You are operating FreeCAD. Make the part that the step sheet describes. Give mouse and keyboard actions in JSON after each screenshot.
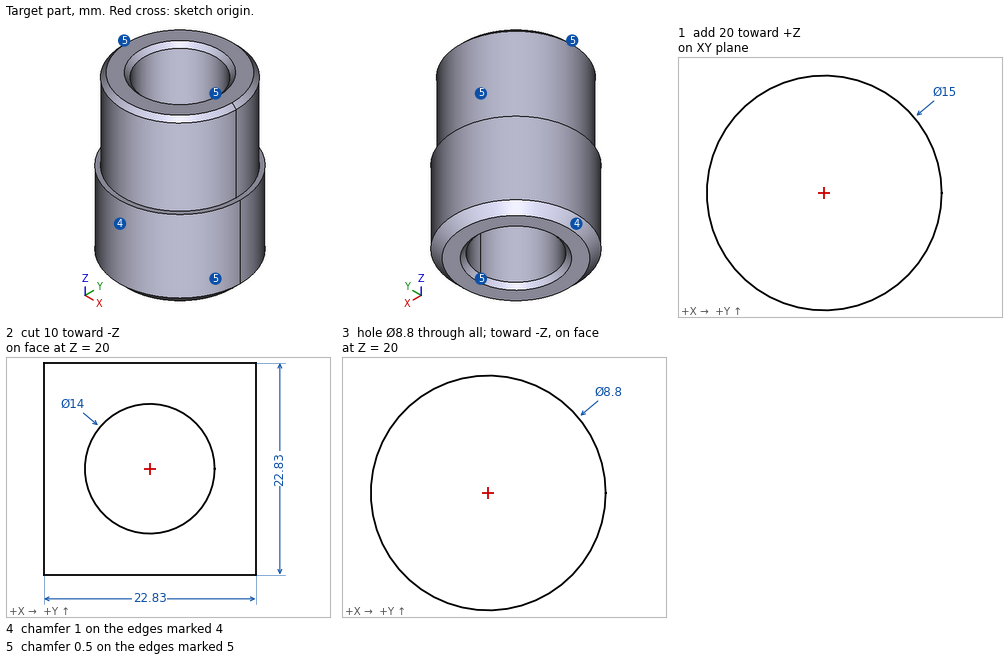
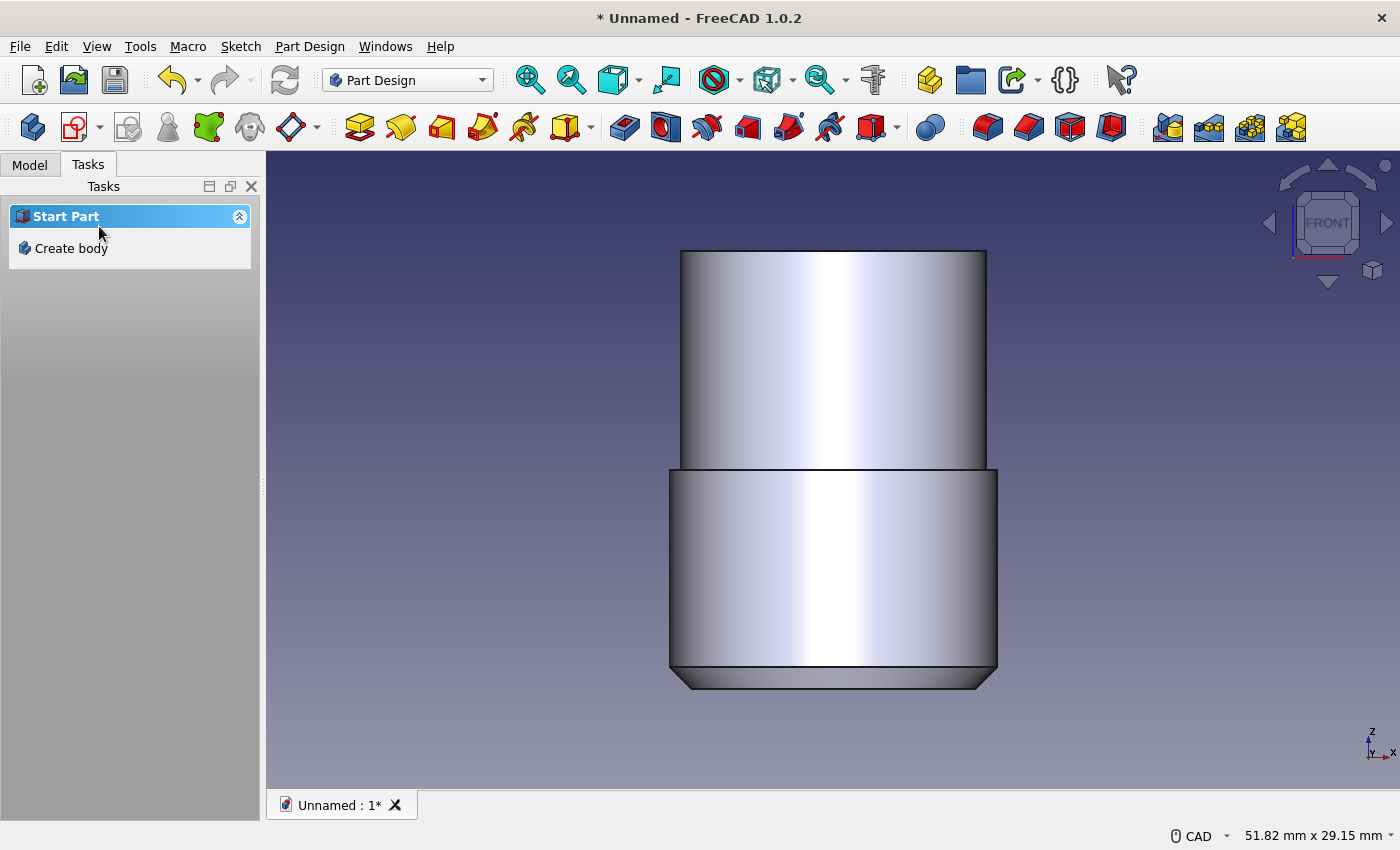
{"action": "left_click", "coordinate": [709, 250]}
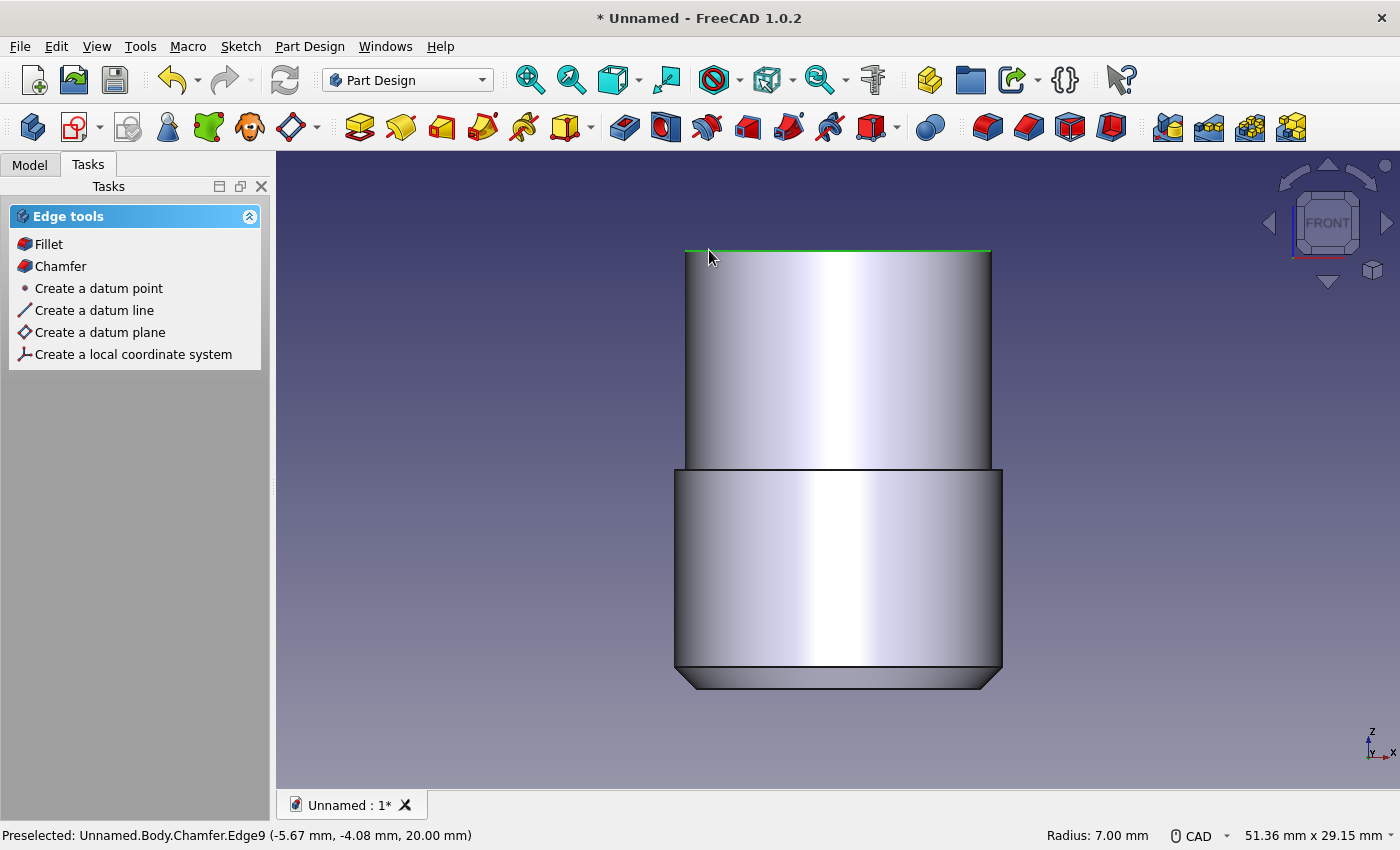
{"action": "key", "text": "0"}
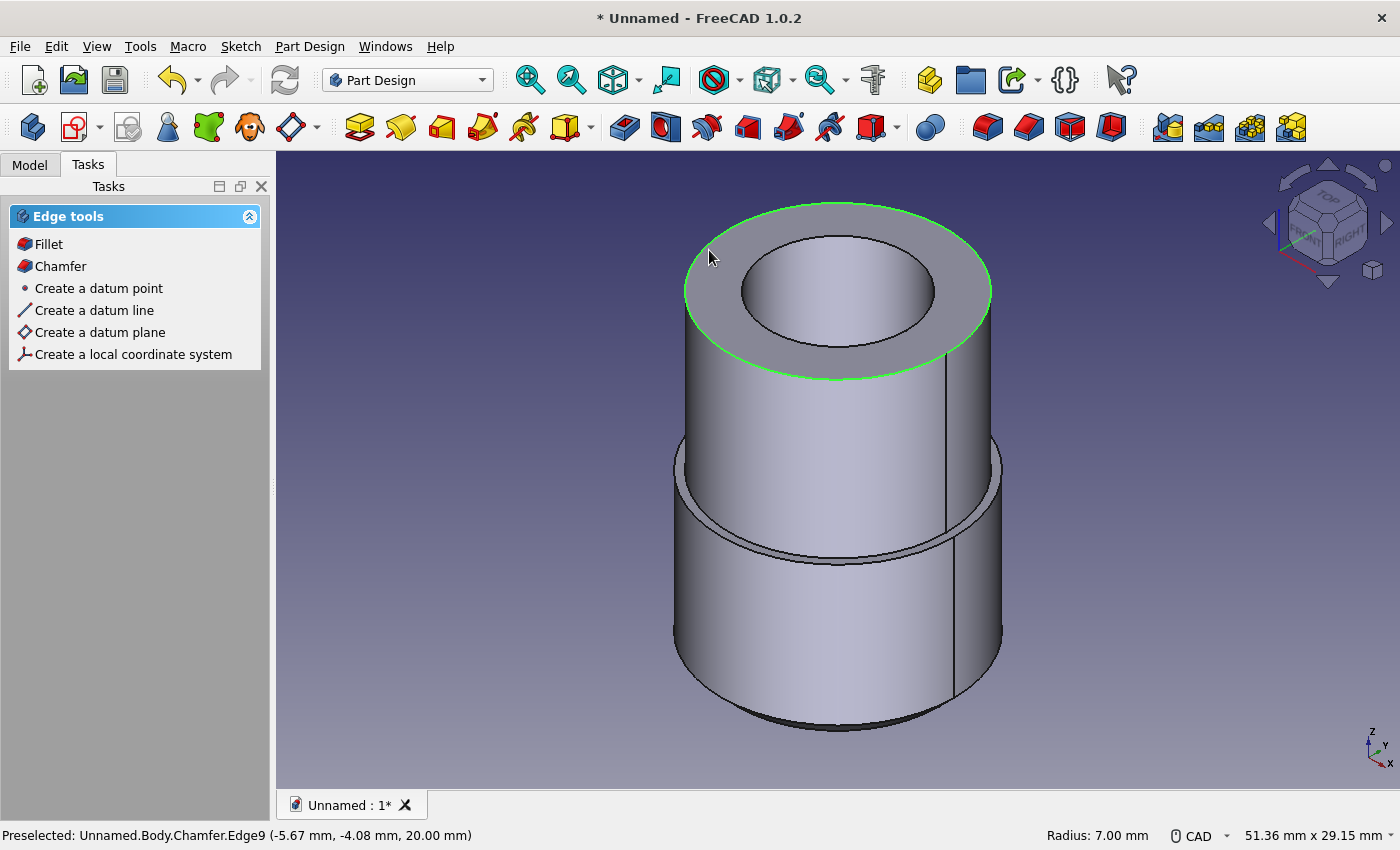
{"action": "left_click", "coordinate": [770, 251], "text": "ctrl"}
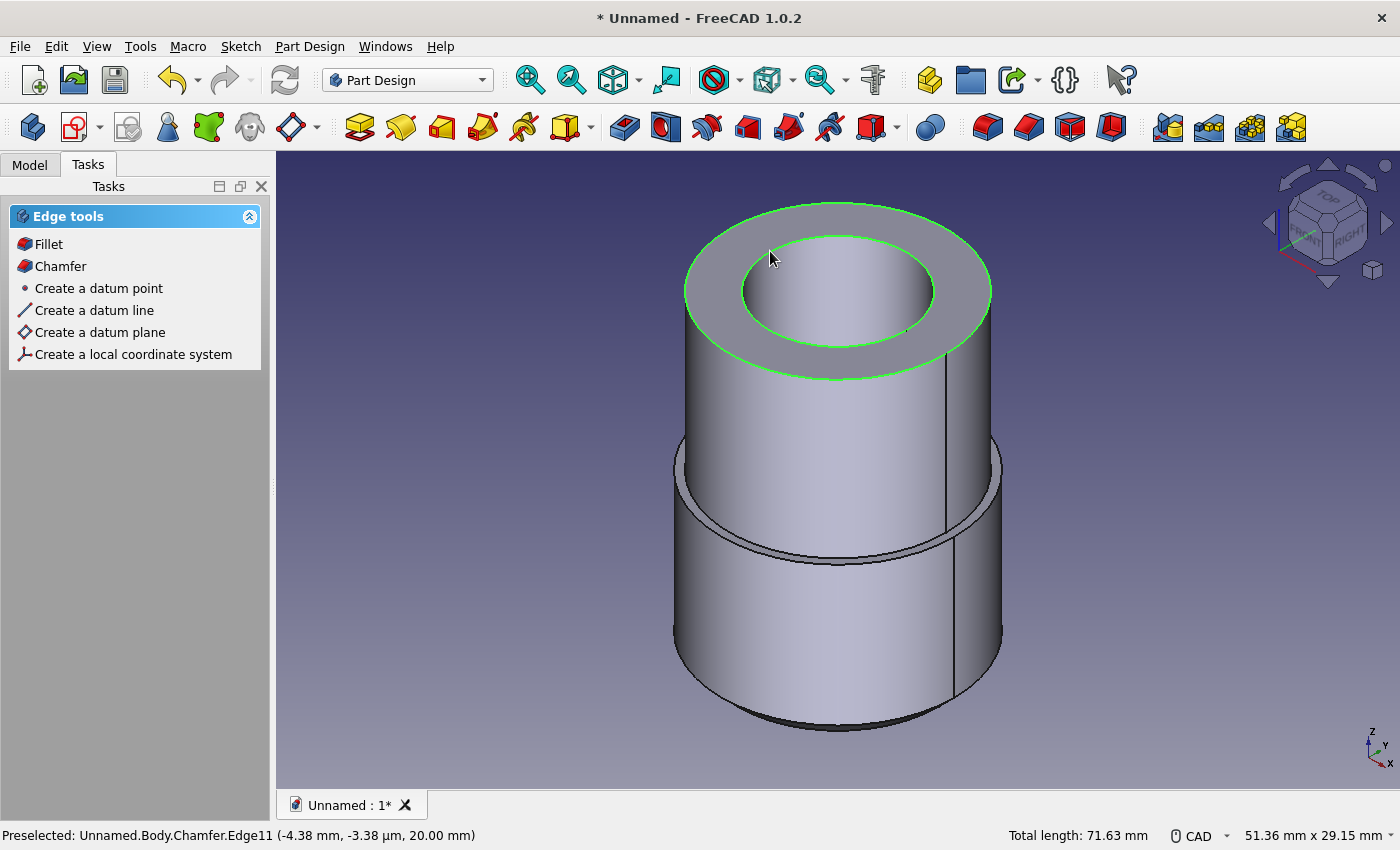
{"action": "key", "text": "2"}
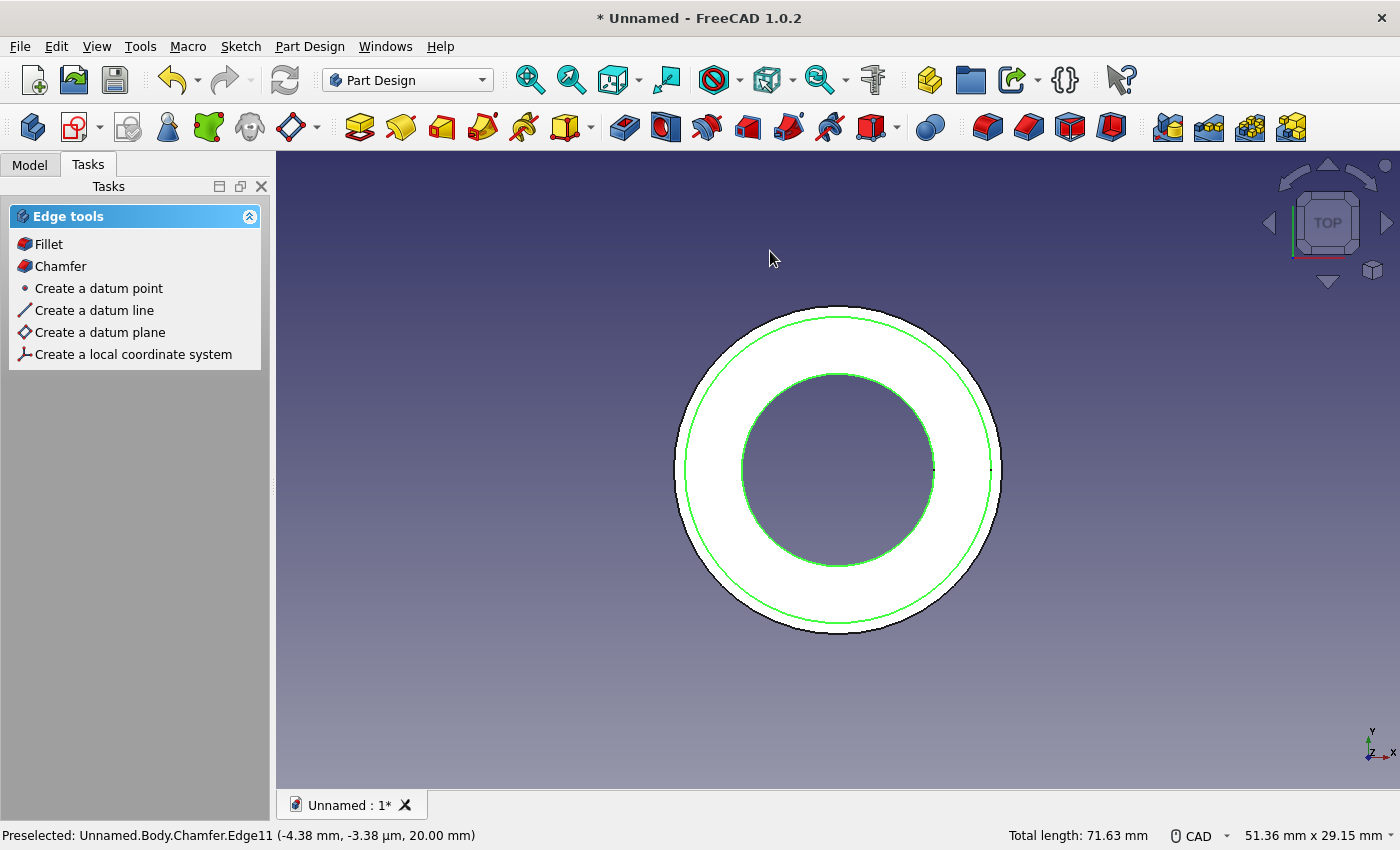
{"action": "key", "text": "1"}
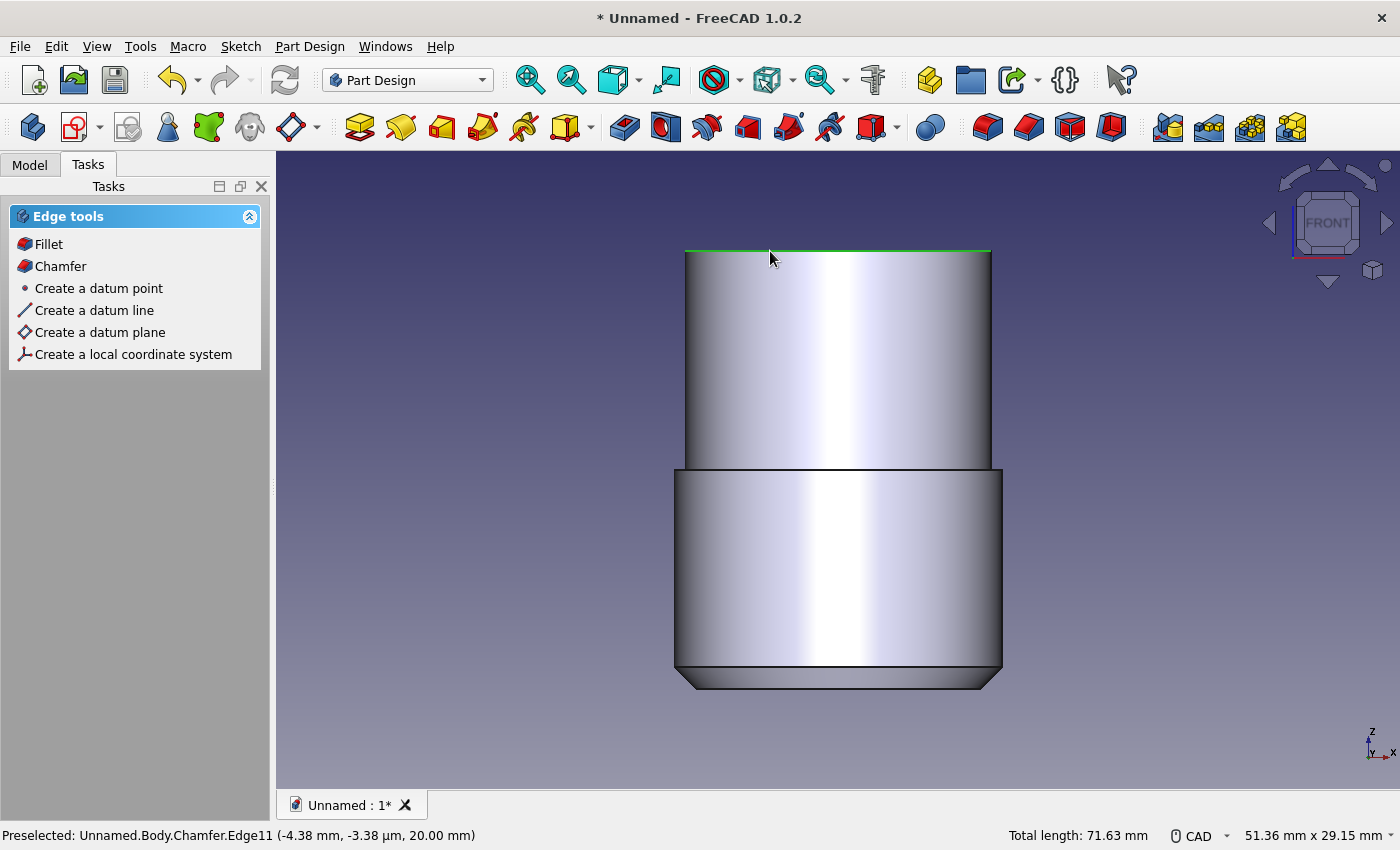
{"action": "key", "text": "3"}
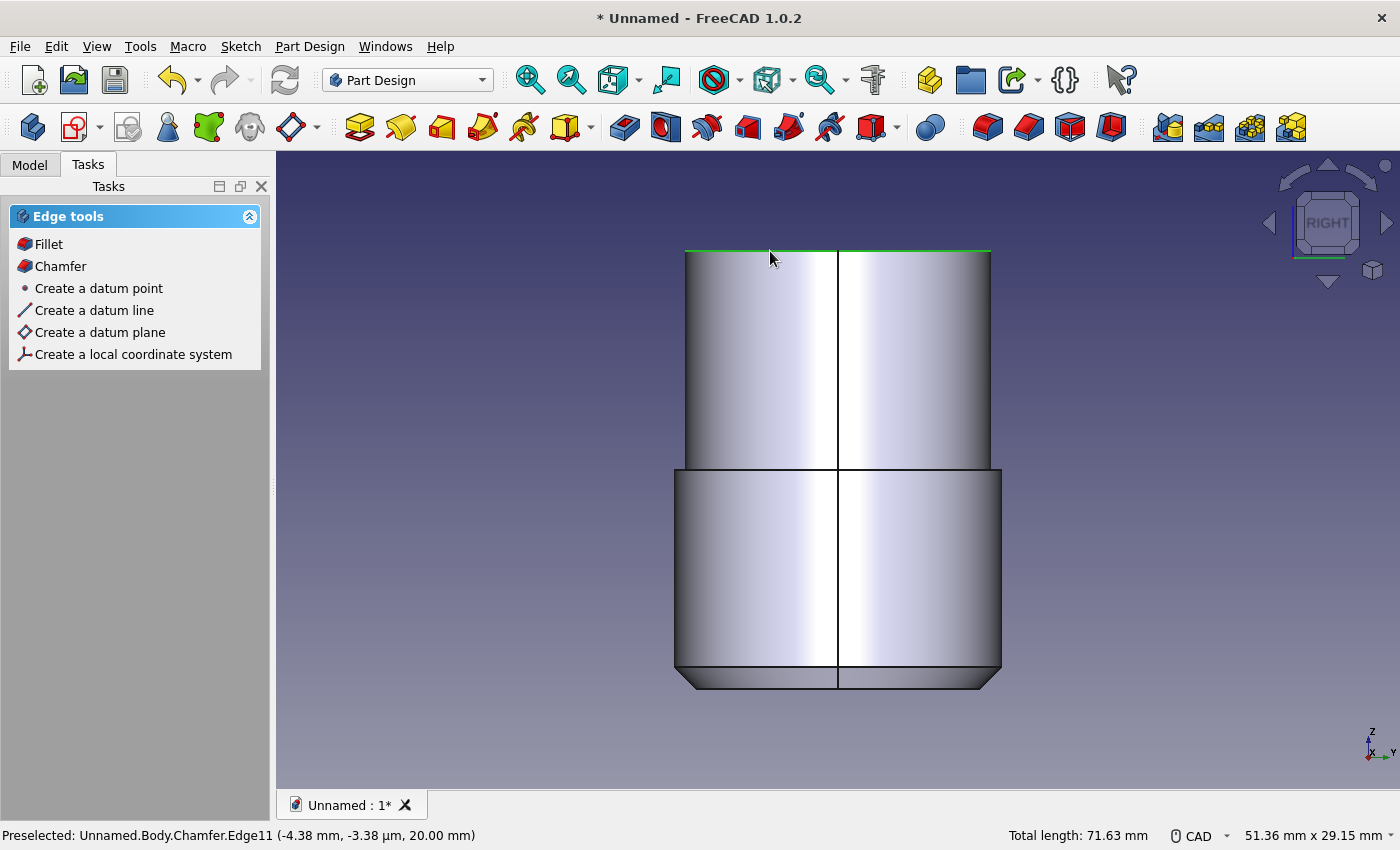
{"action": "key", "text": "5"}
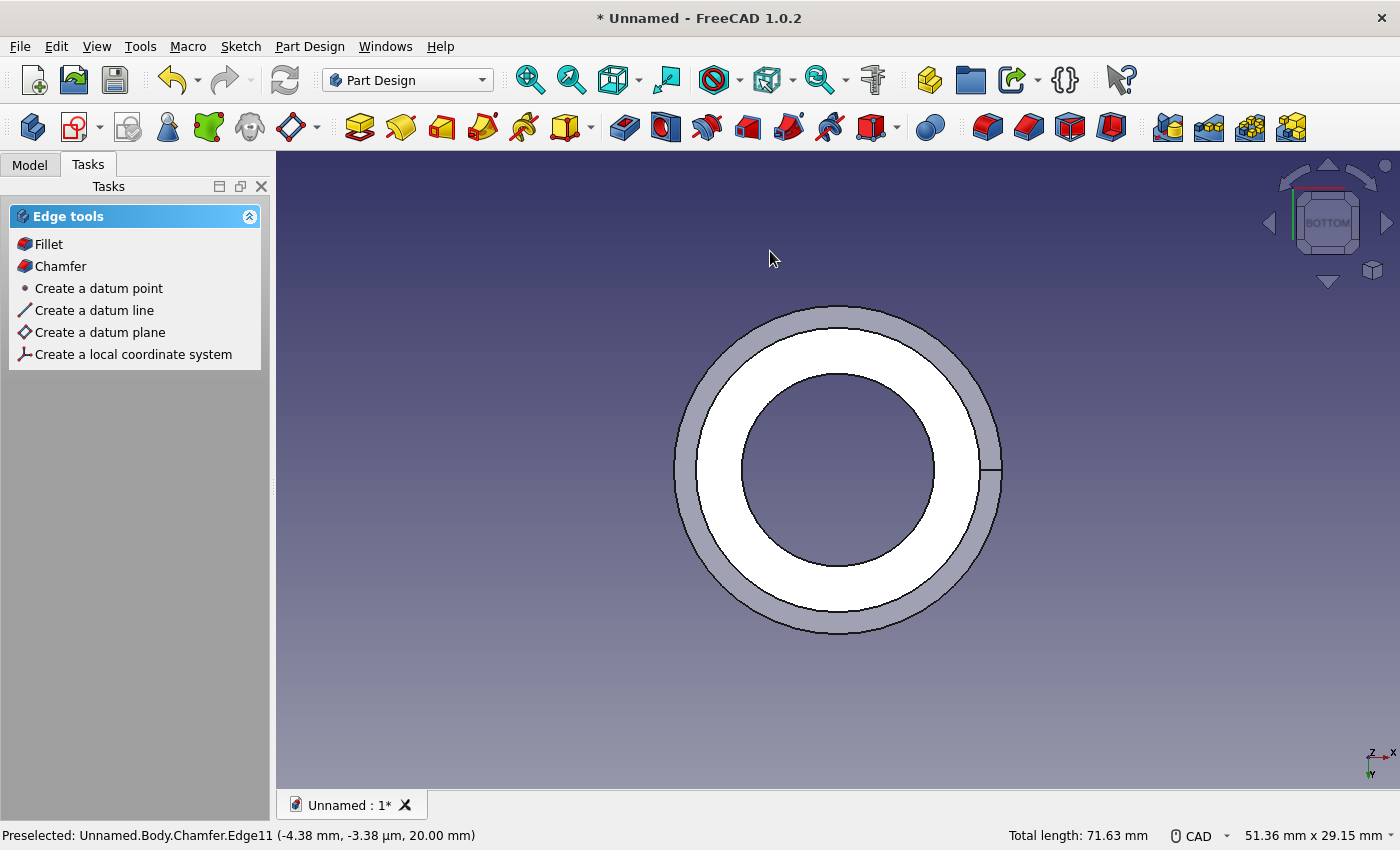
{"action": "left_click", "coordinate": [742, 469], "text": "ctrl"}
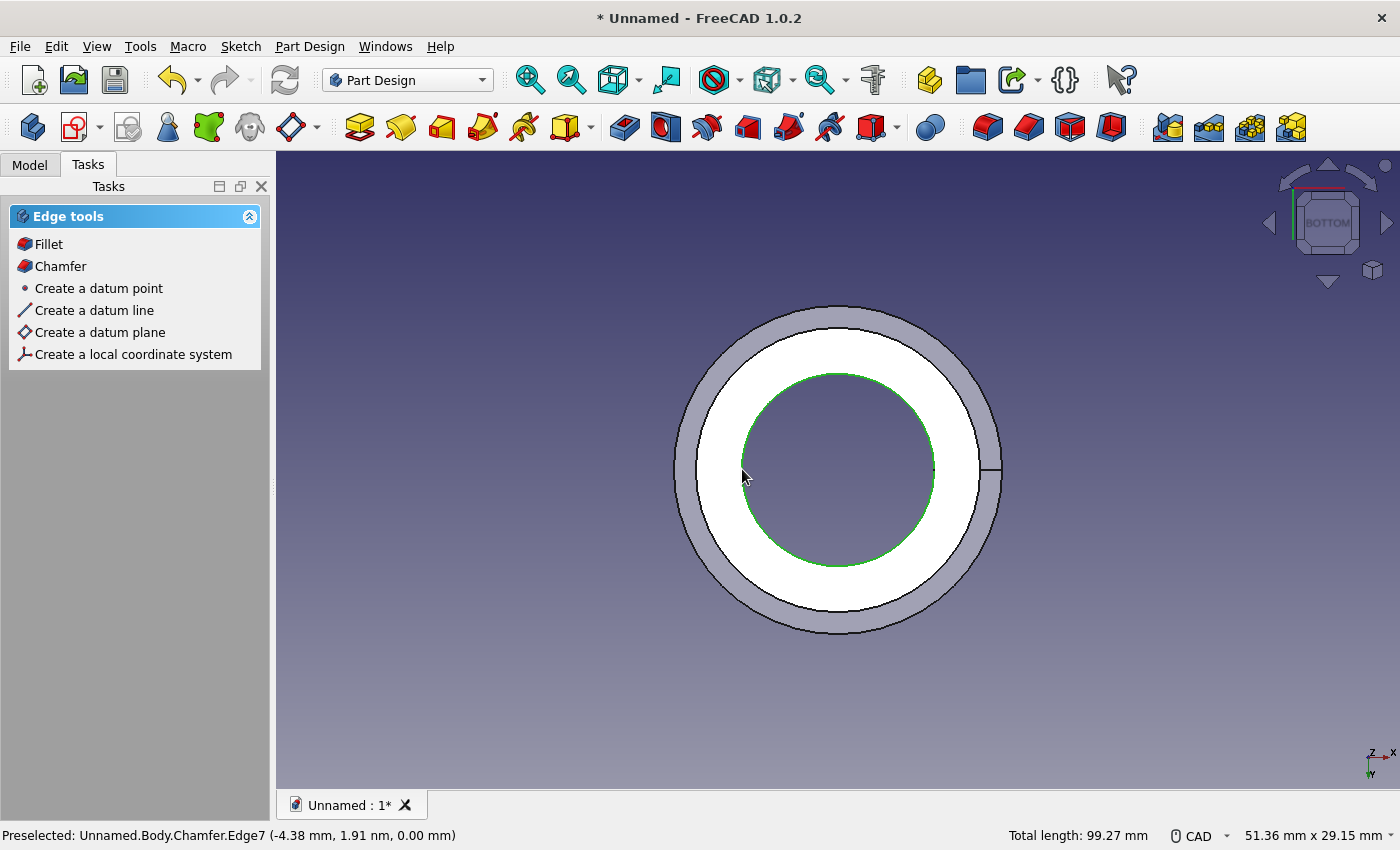
{"action": "left_click", "coordinate": [1029, 128]}